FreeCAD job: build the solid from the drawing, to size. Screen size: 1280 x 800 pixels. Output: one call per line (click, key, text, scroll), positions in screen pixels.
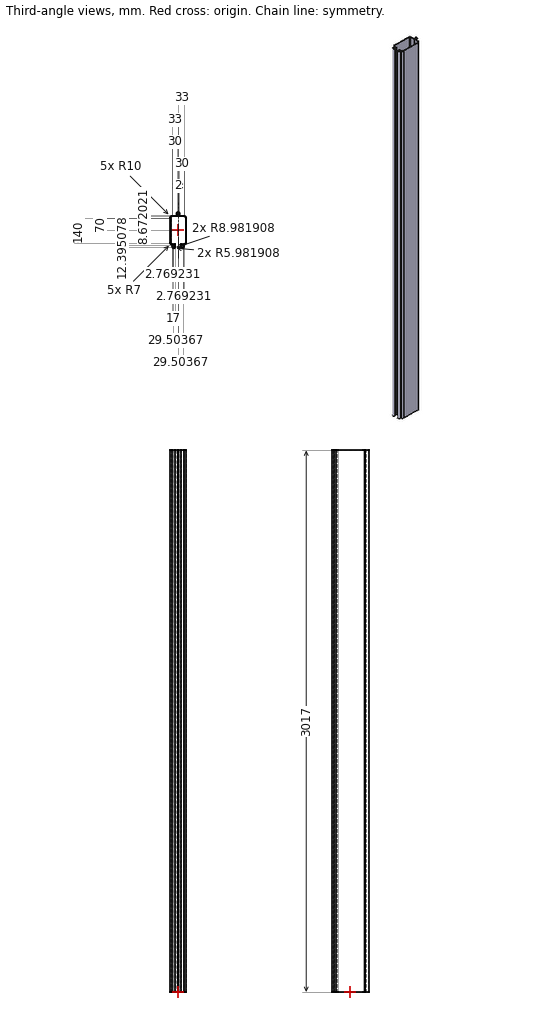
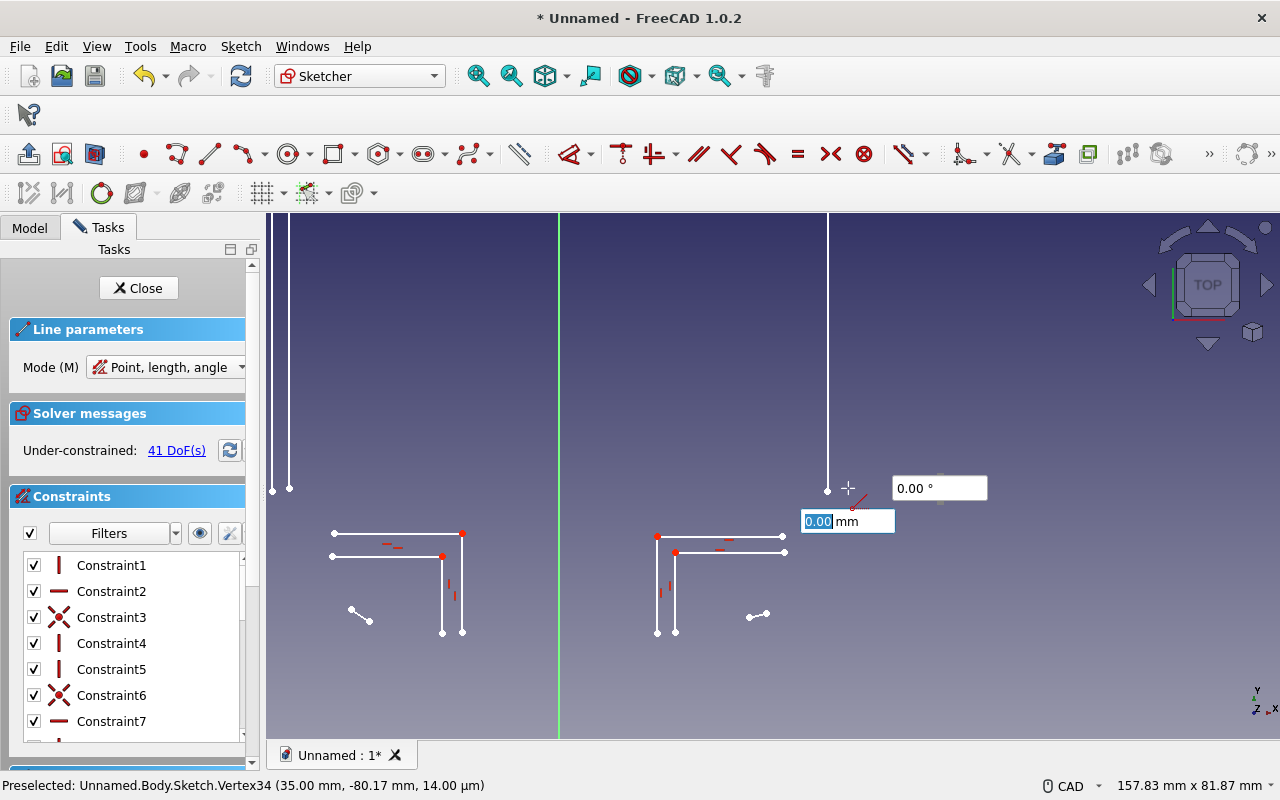
scroll(752, 621, down, 7)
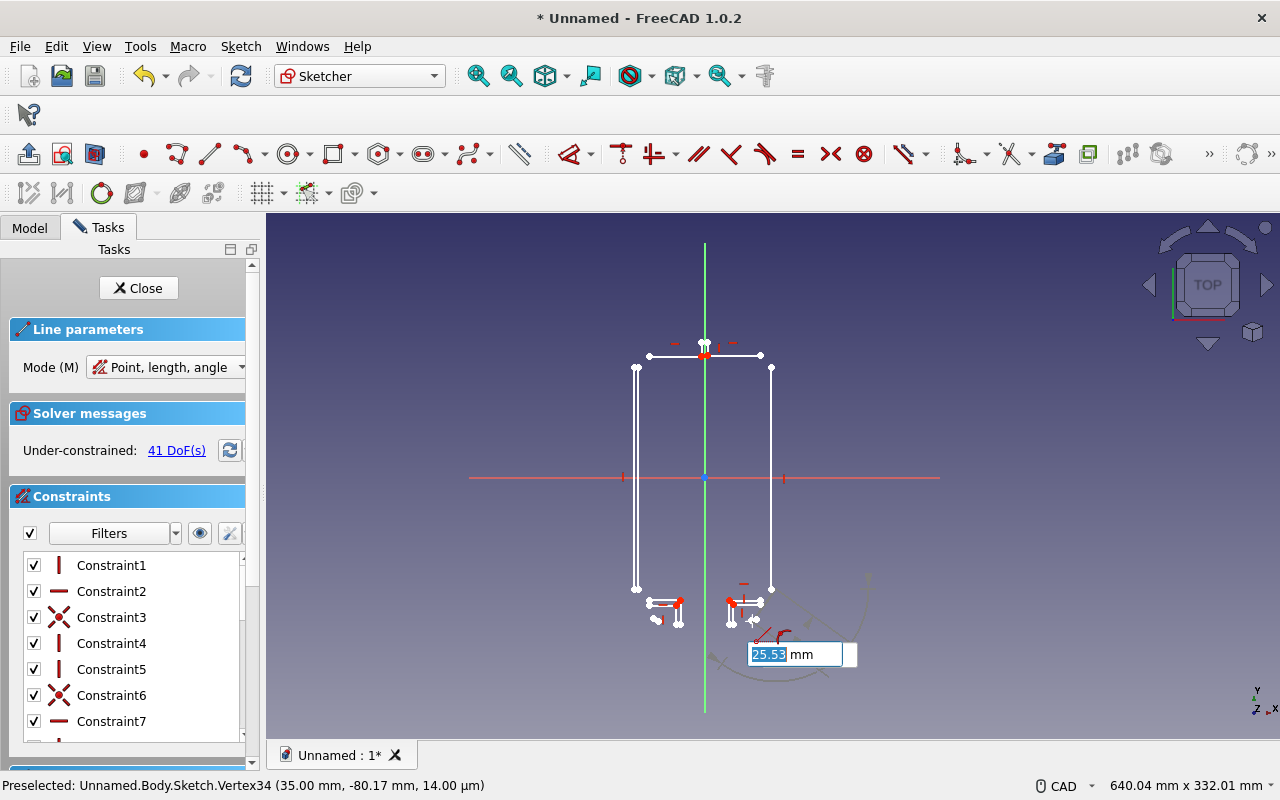
scroll(776, 367, up, 7)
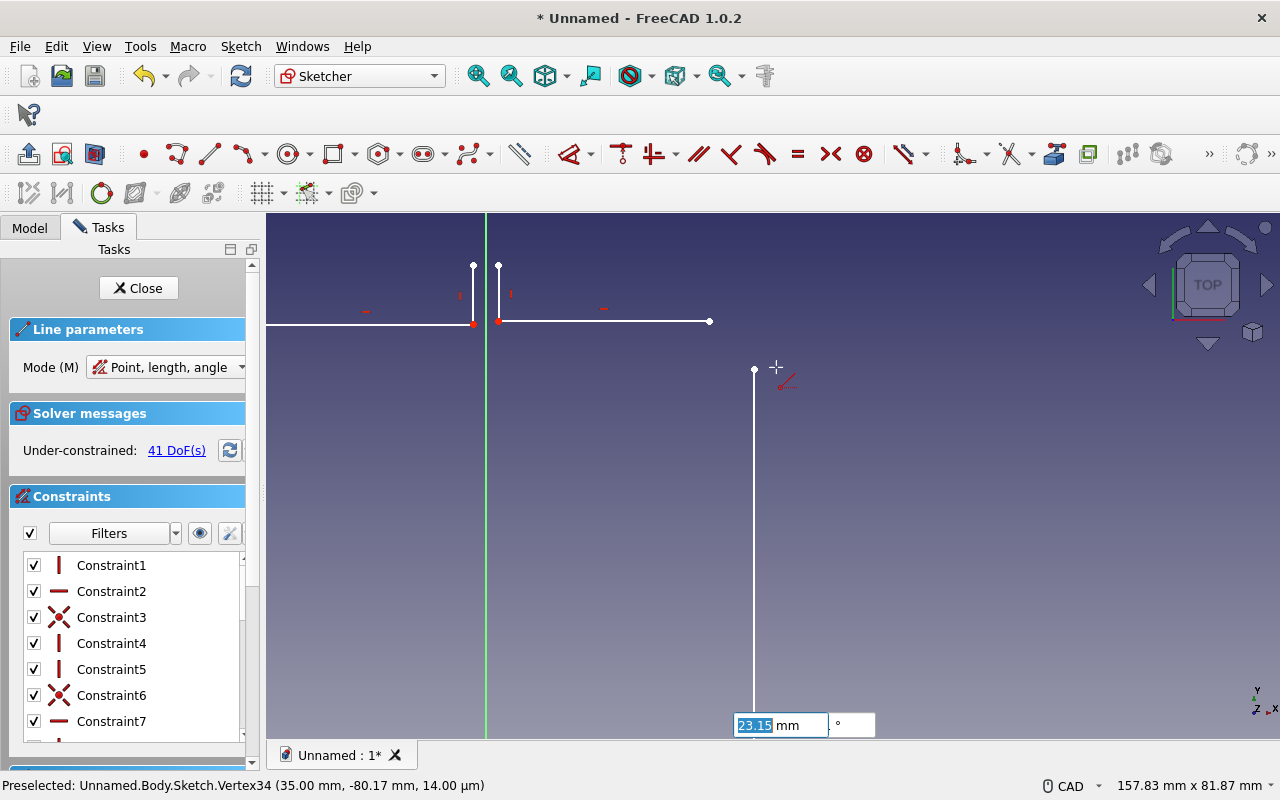
click(775, 366)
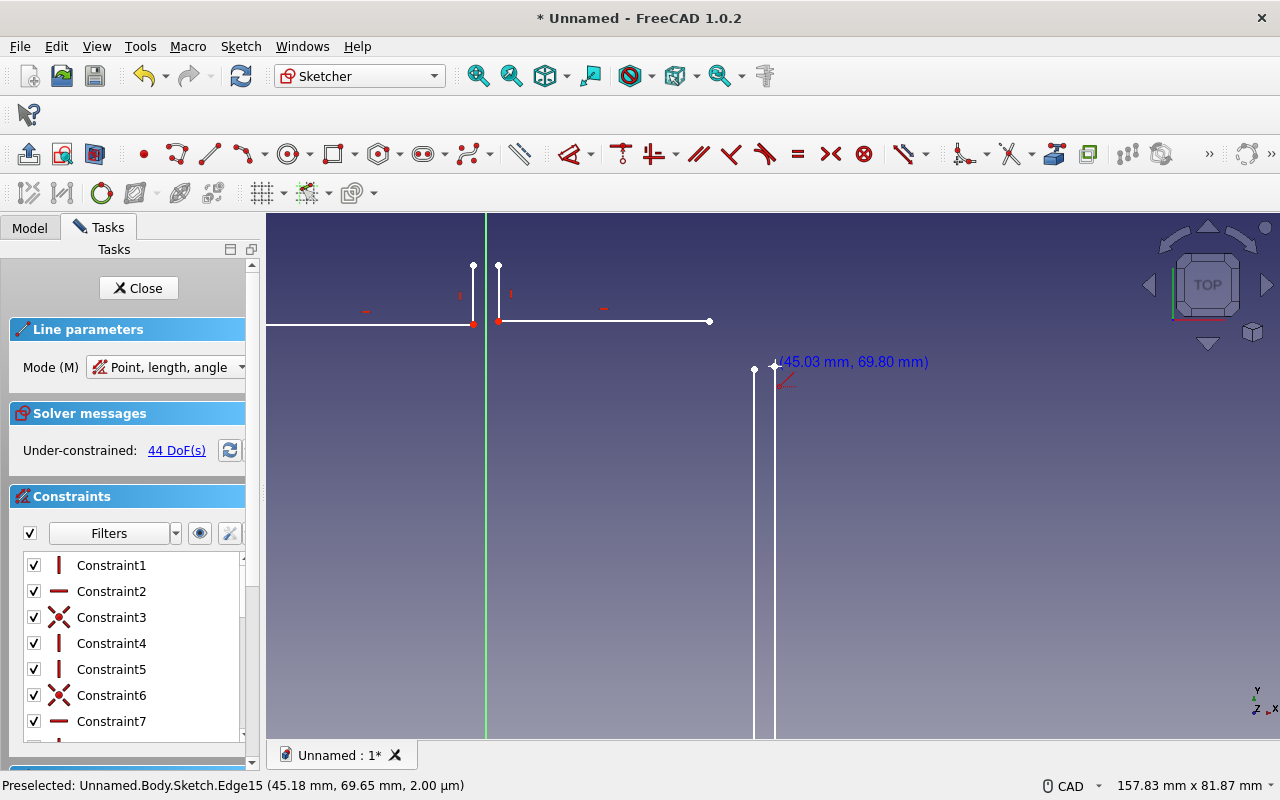
click(177, 154)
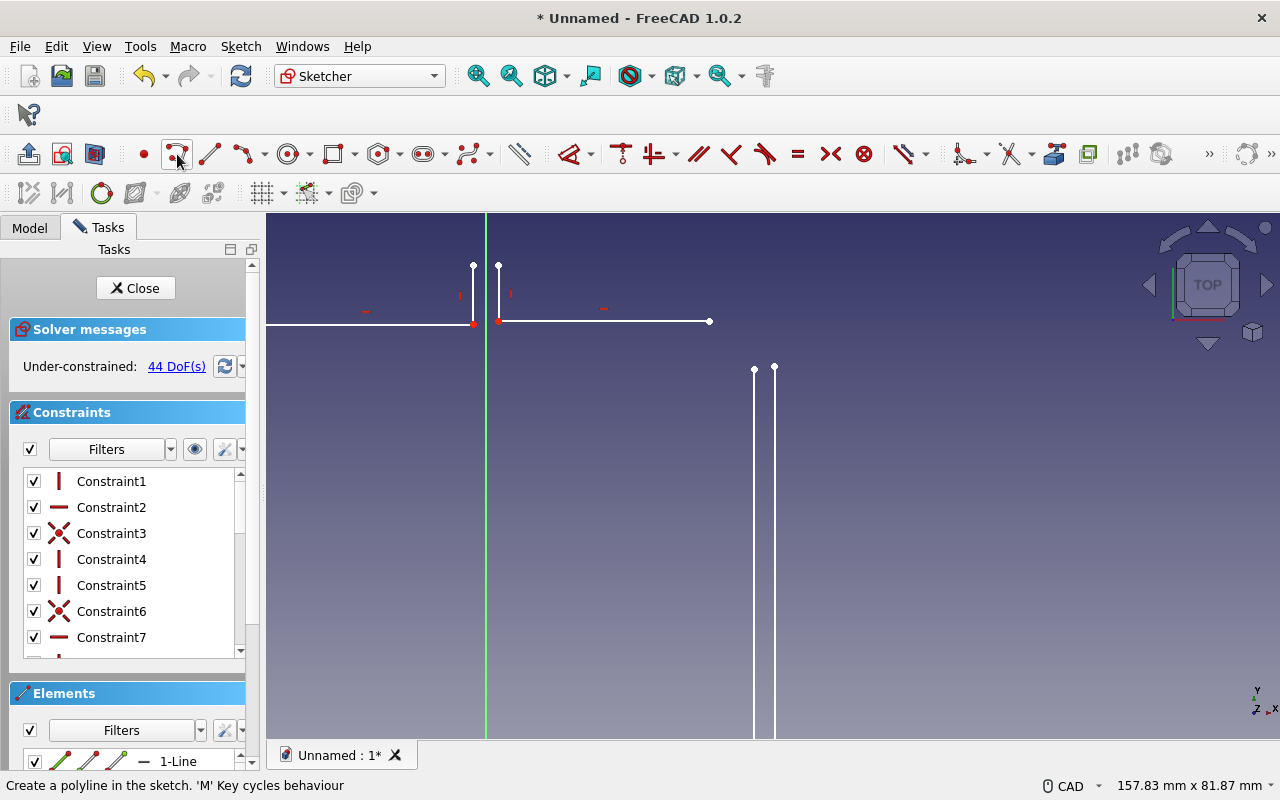
click(711, 301)
click(518, 301)
click(518, 278)
right_click(518, 278)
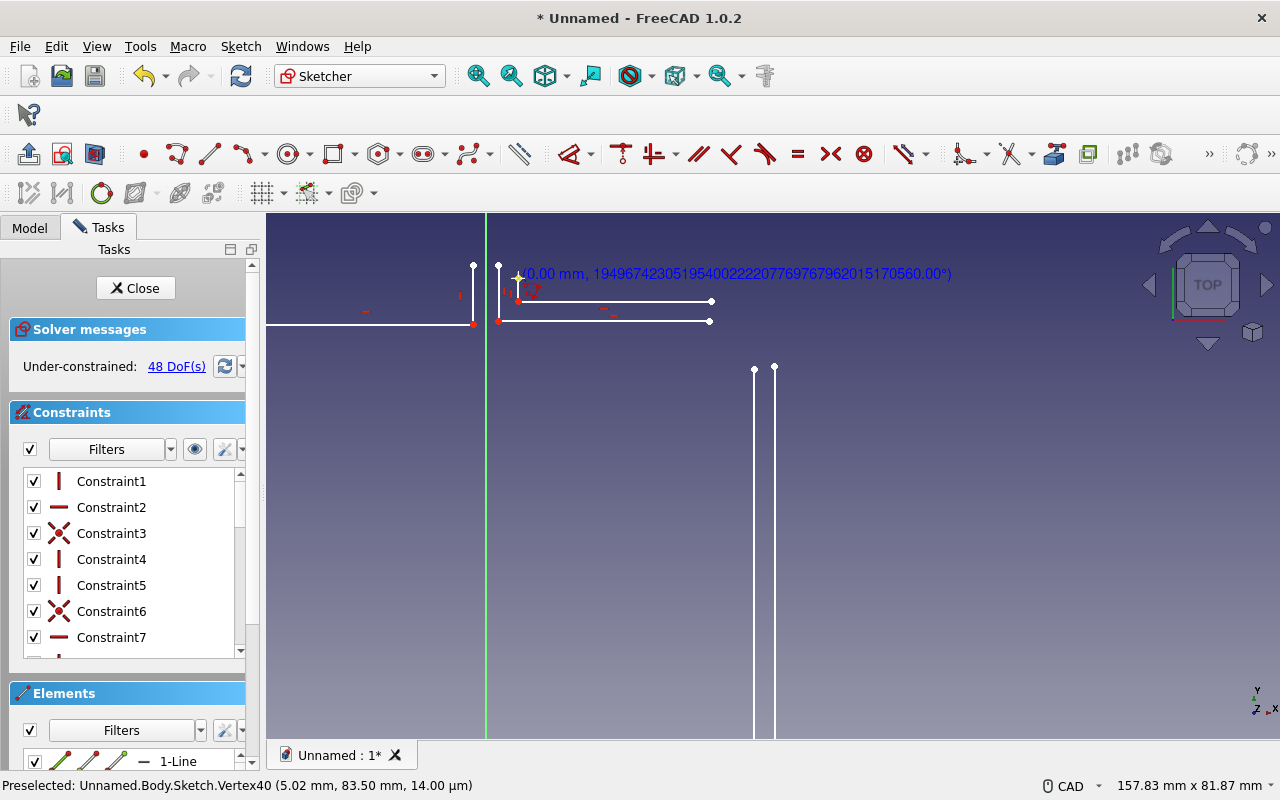
click(454, 278)
click(454, 301)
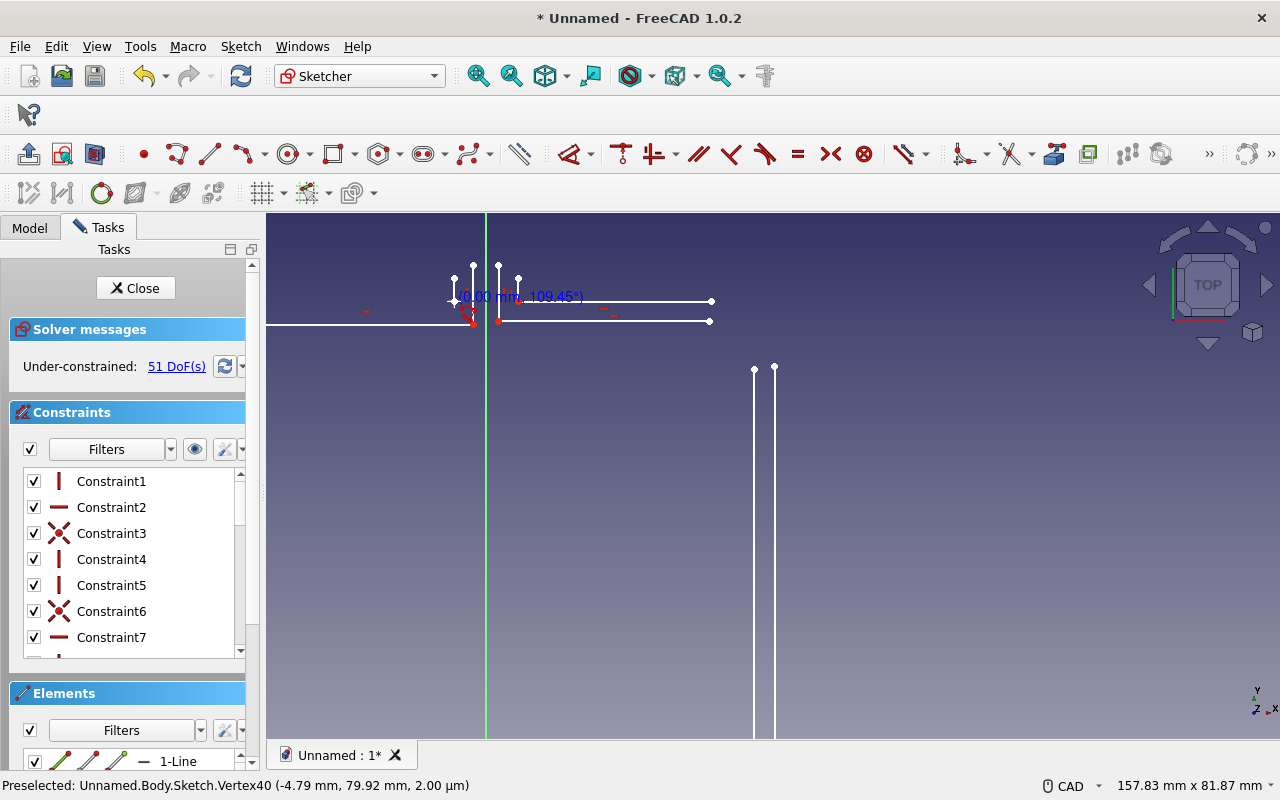
scroll(776, 366, down, 7)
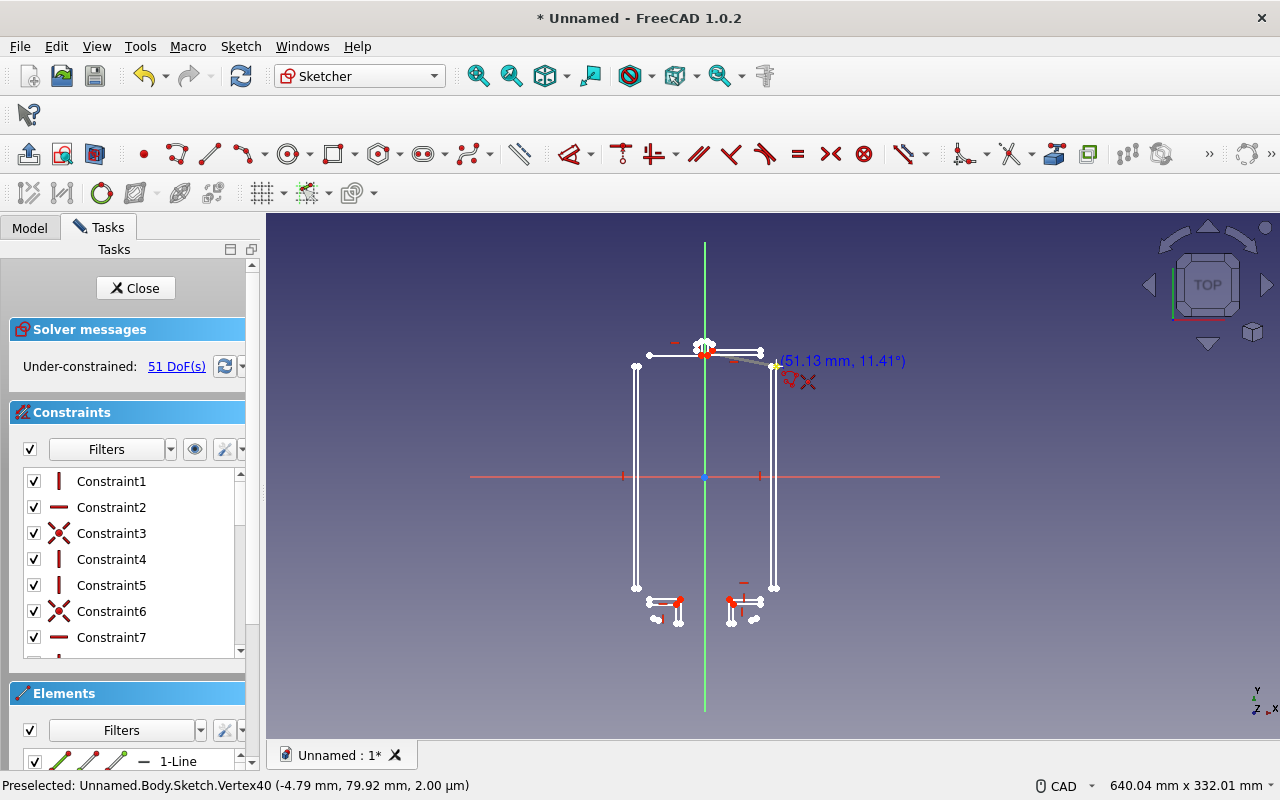
scroll(649, 350, up, 7)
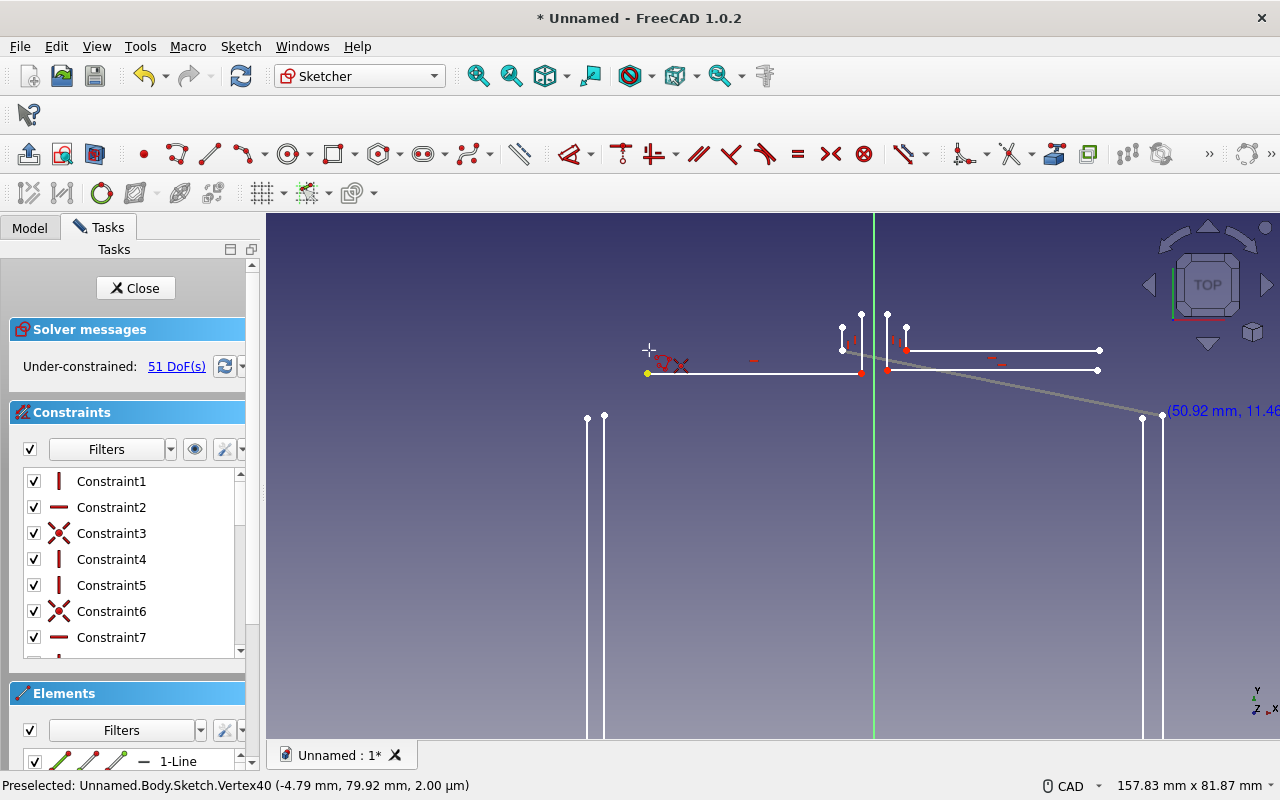
click(649, 350)
right_click(649, 350)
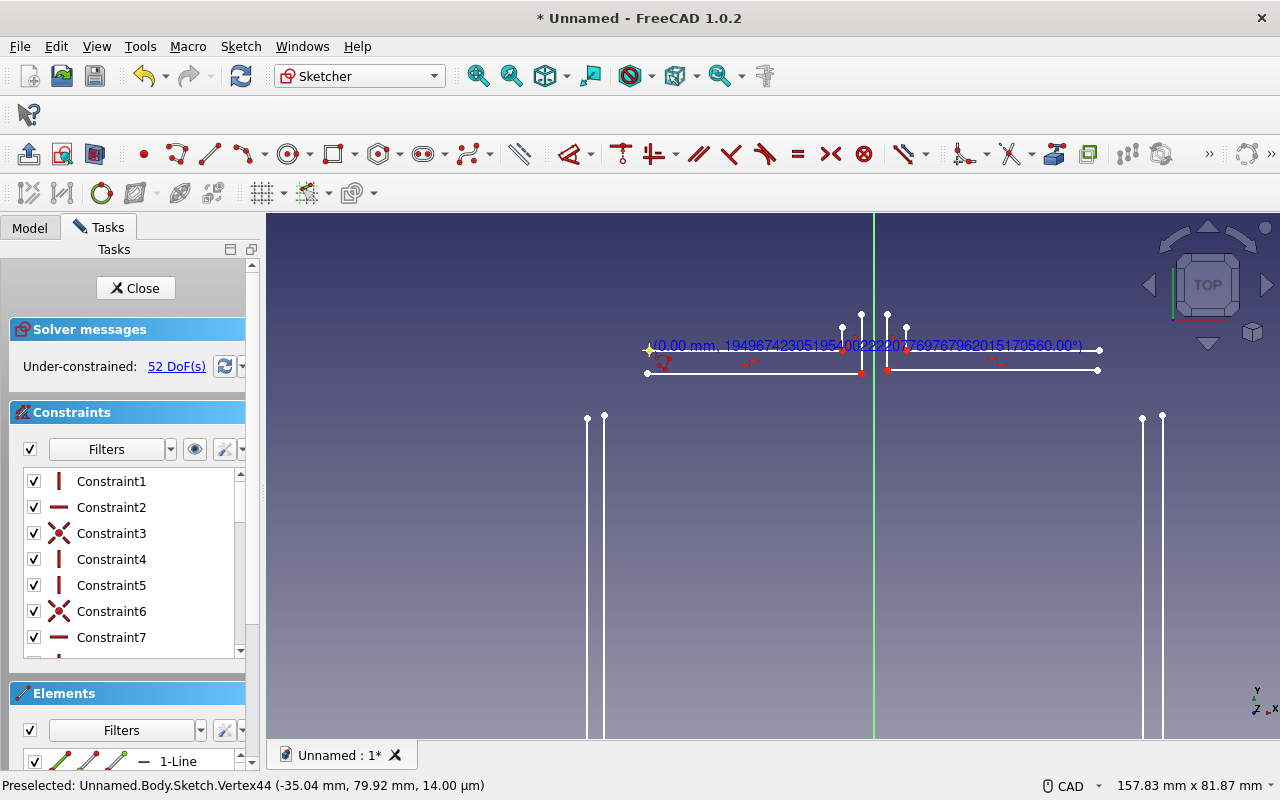
click(242, 154)